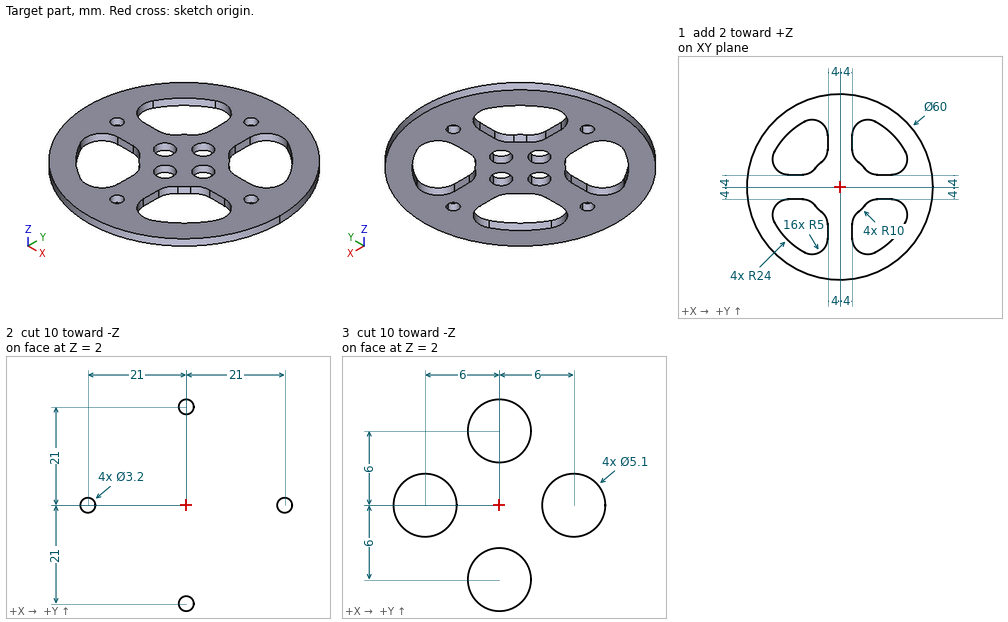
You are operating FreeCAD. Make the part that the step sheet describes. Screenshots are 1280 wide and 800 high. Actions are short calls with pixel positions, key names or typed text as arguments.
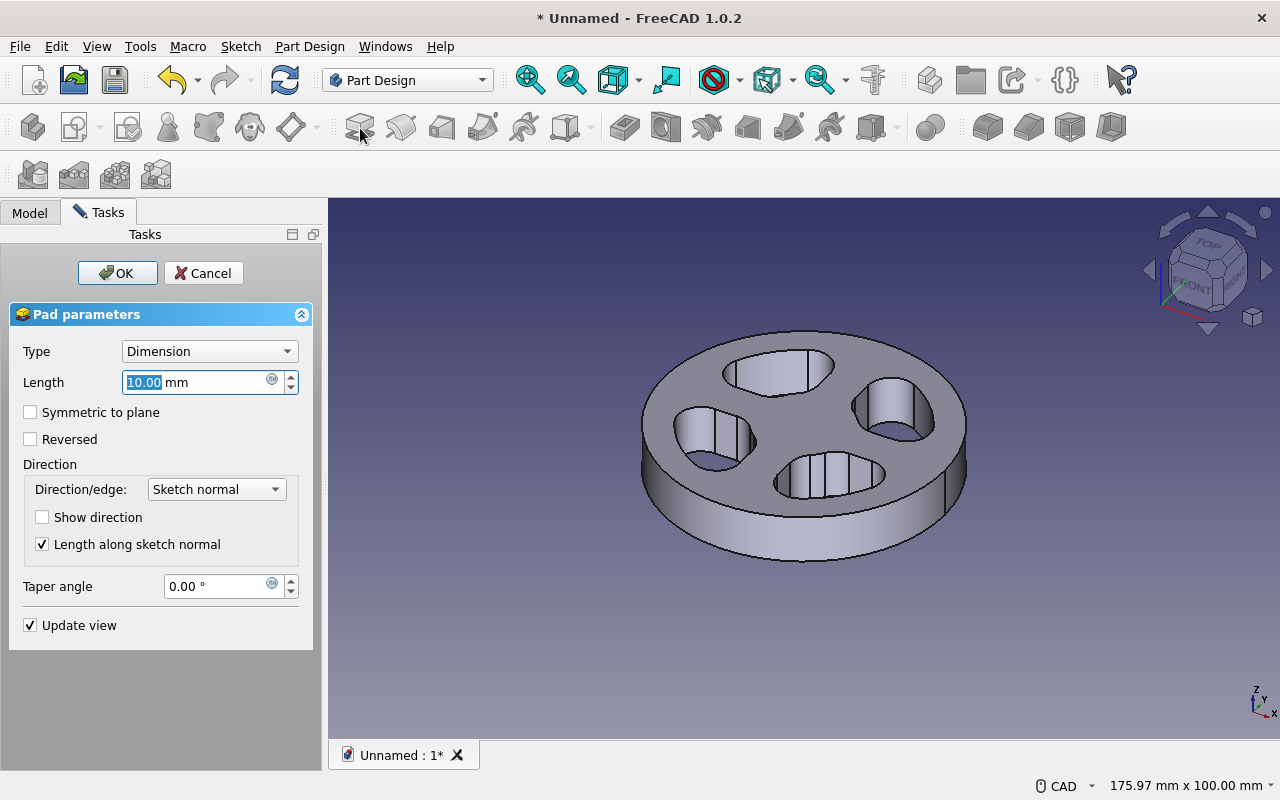
text(2)
key(Tab)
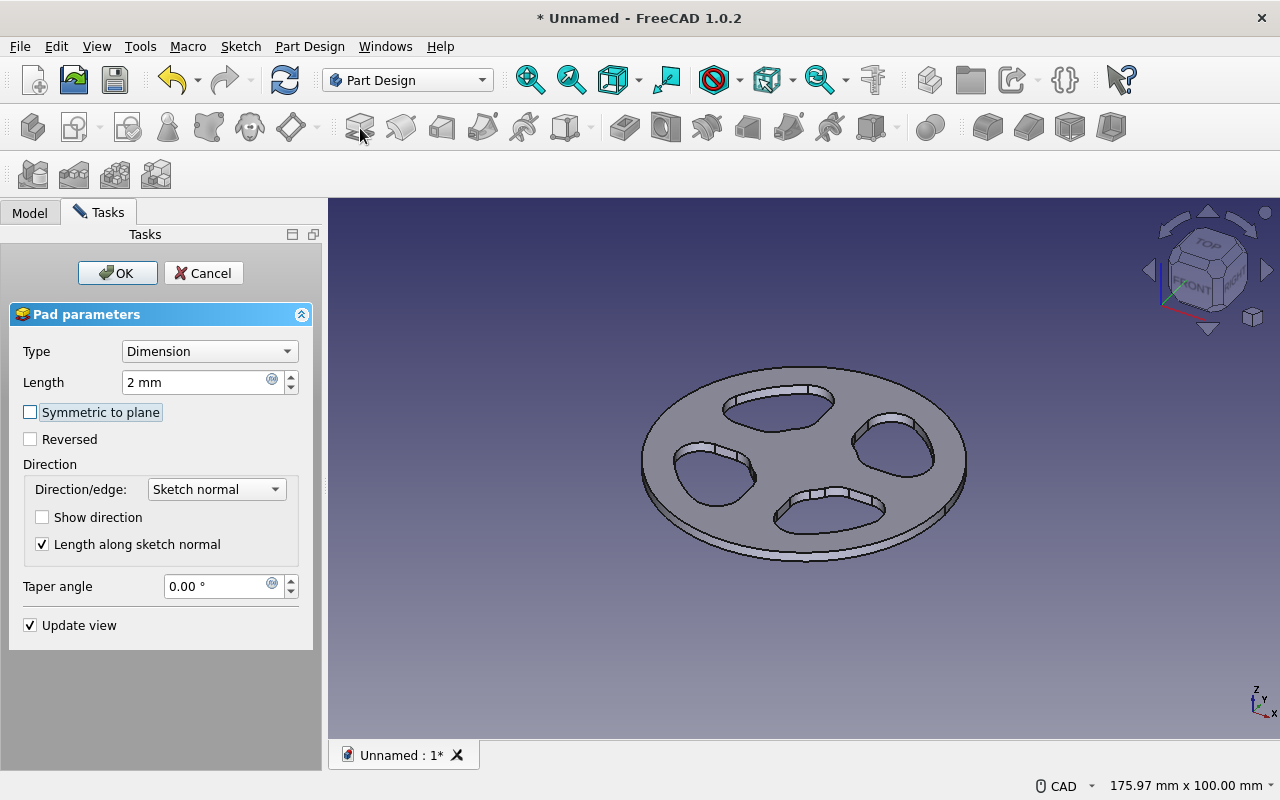
click(118, 273)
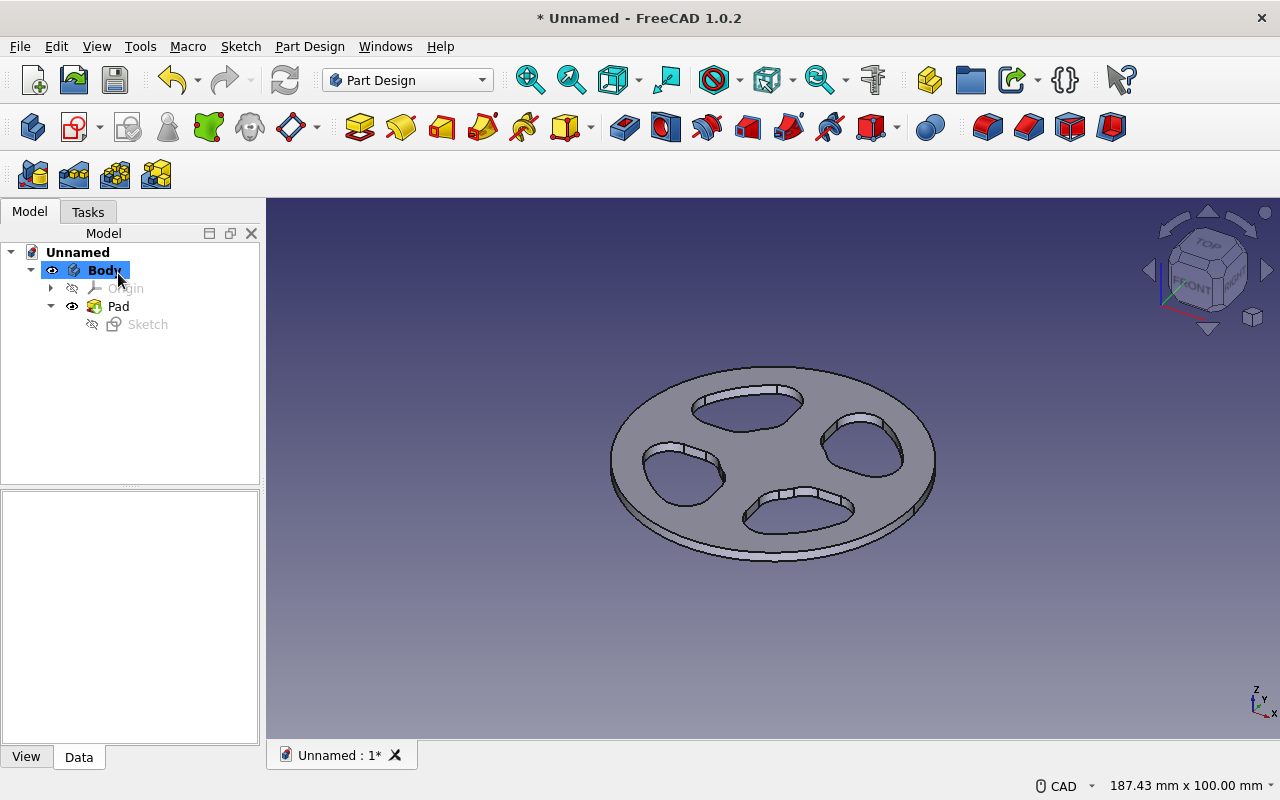
click(773, 459)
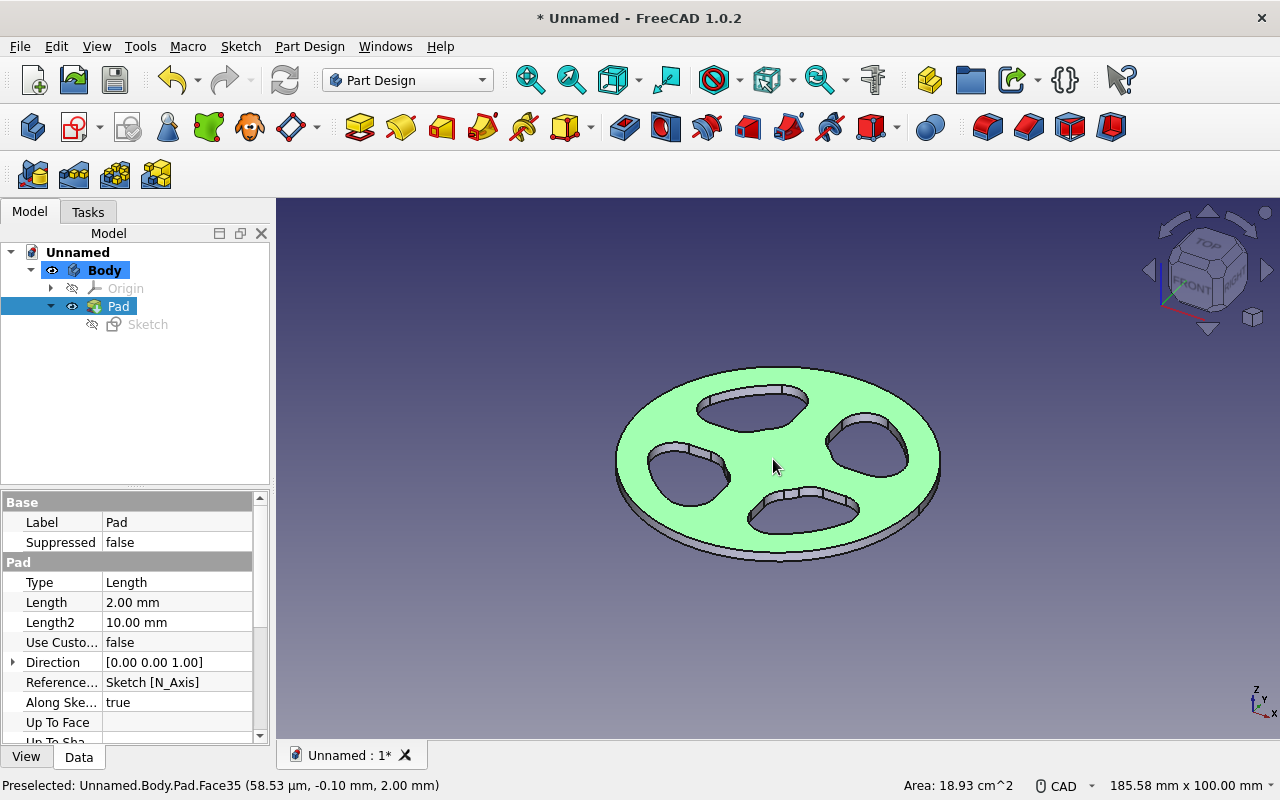
click(74, 128)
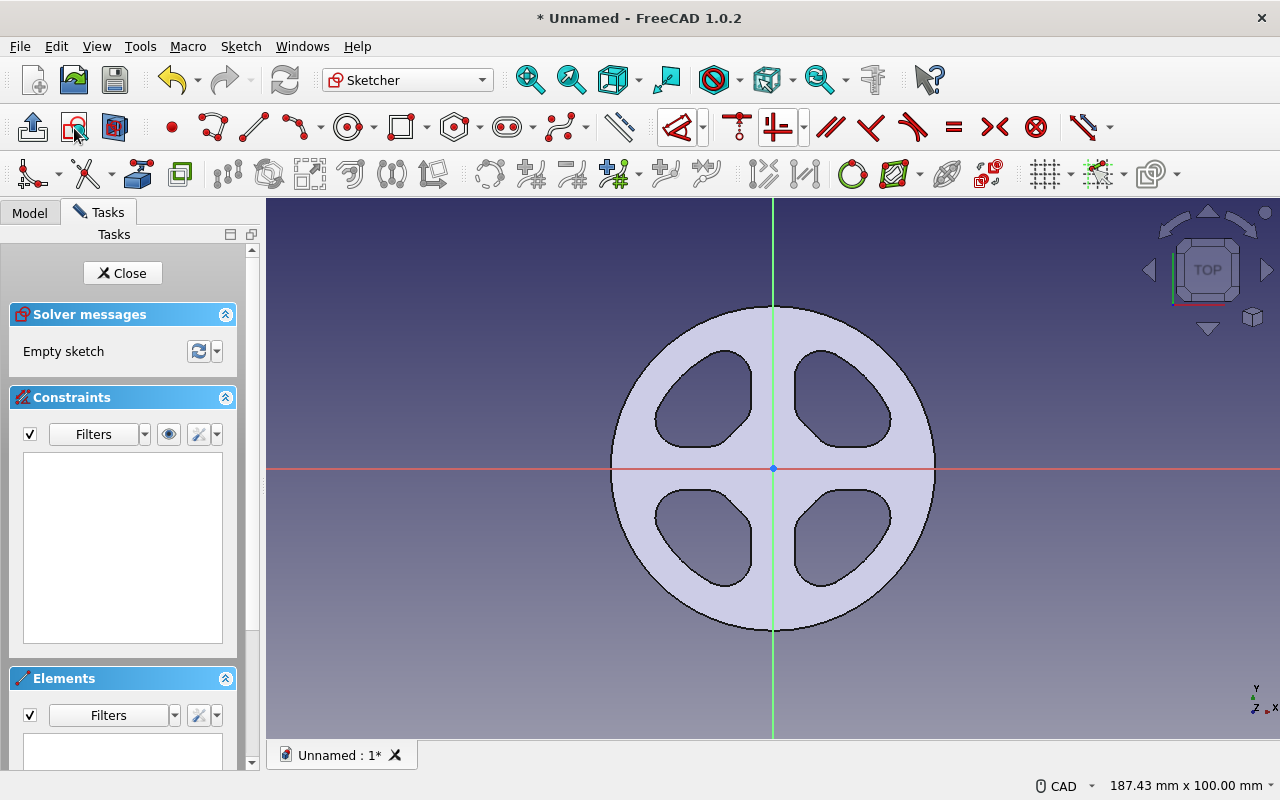
scroll(912, 469, up, 2)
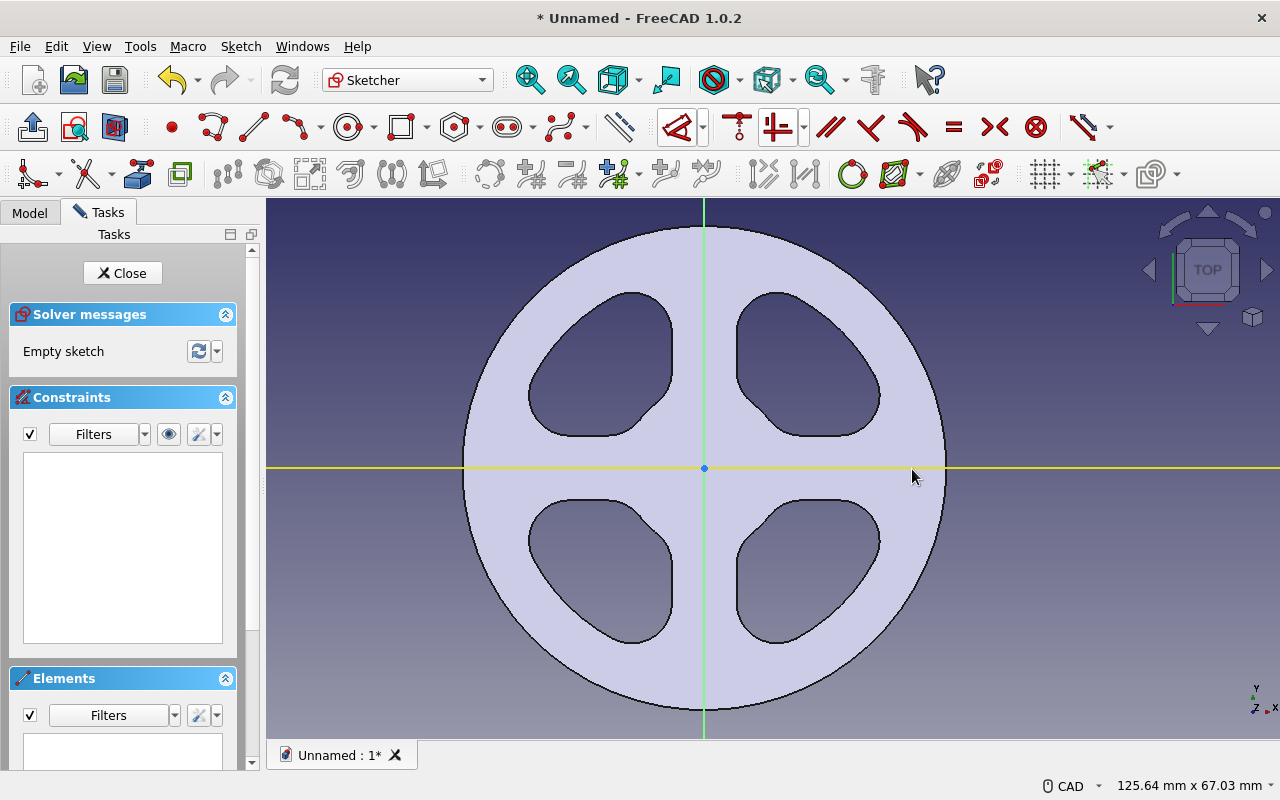
click(348, 128)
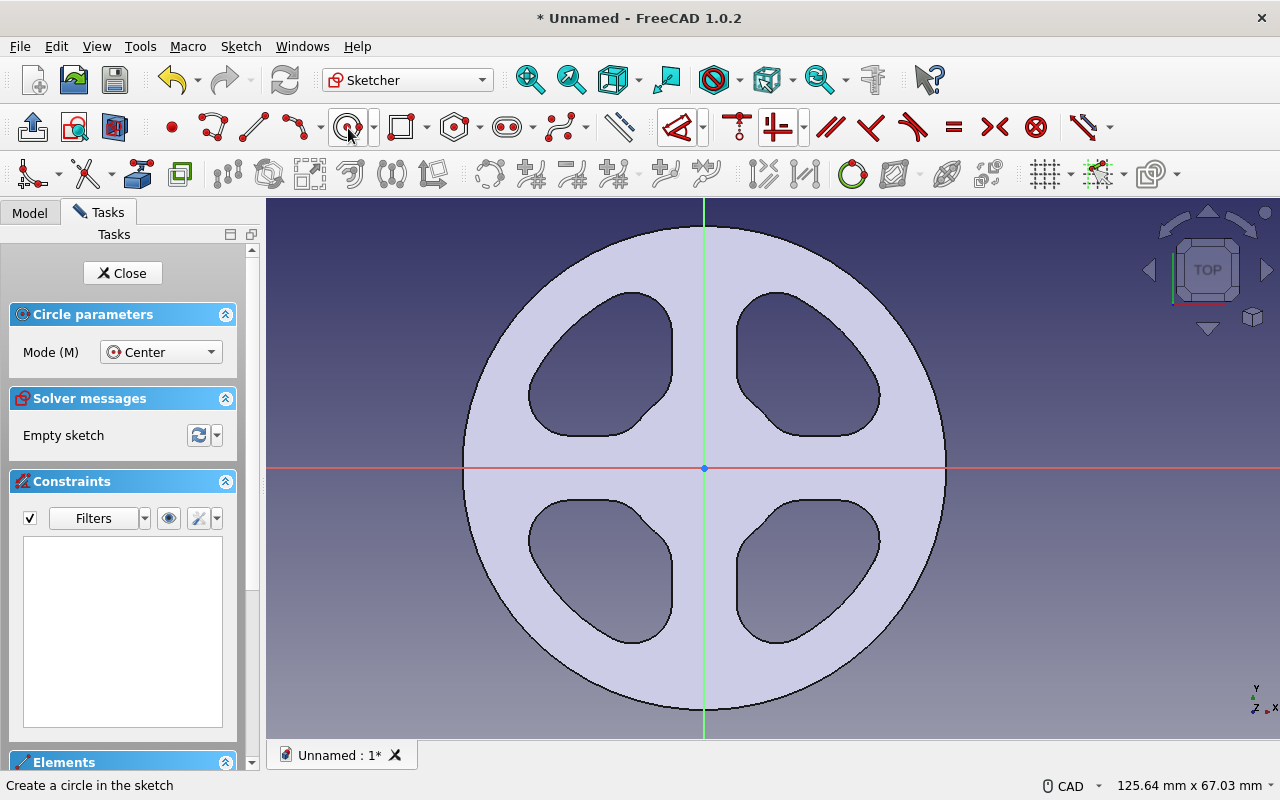
scroll(535, 468, up, 3)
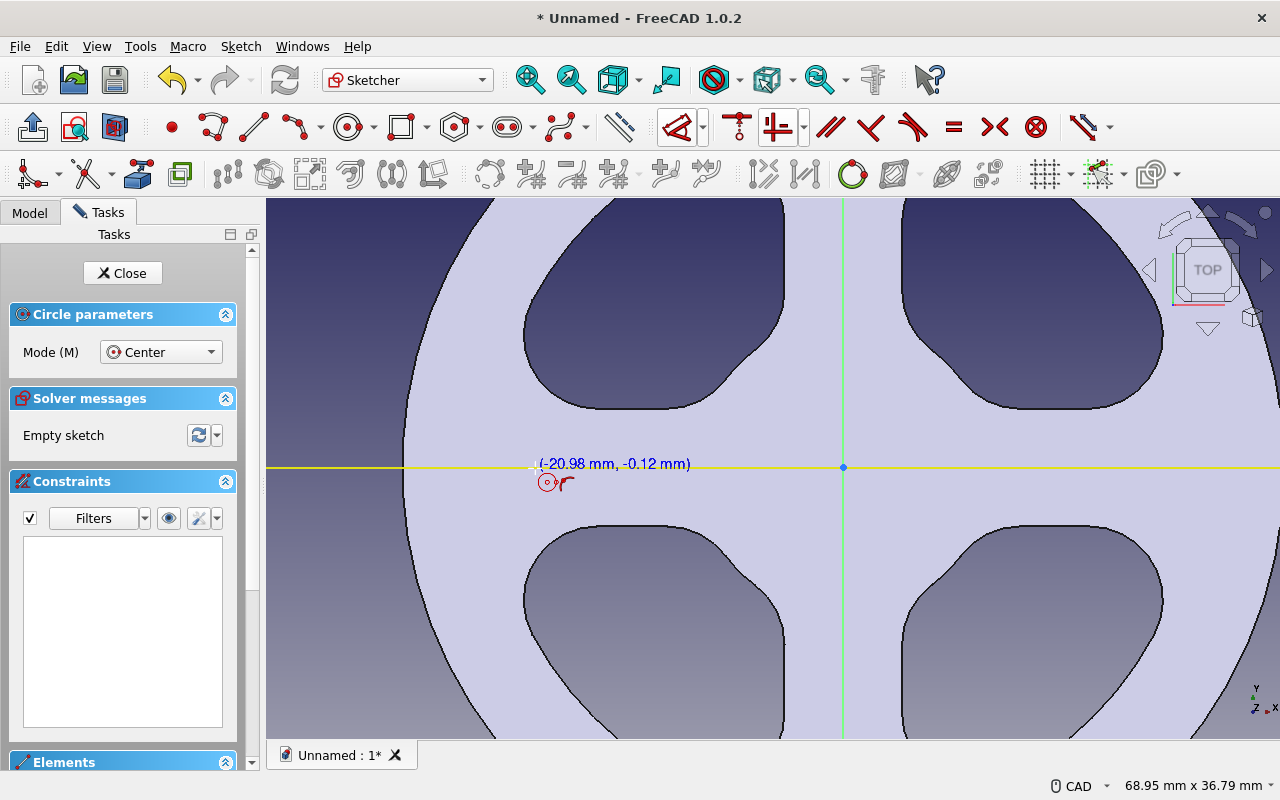
click(534, 468)
move(551, 451)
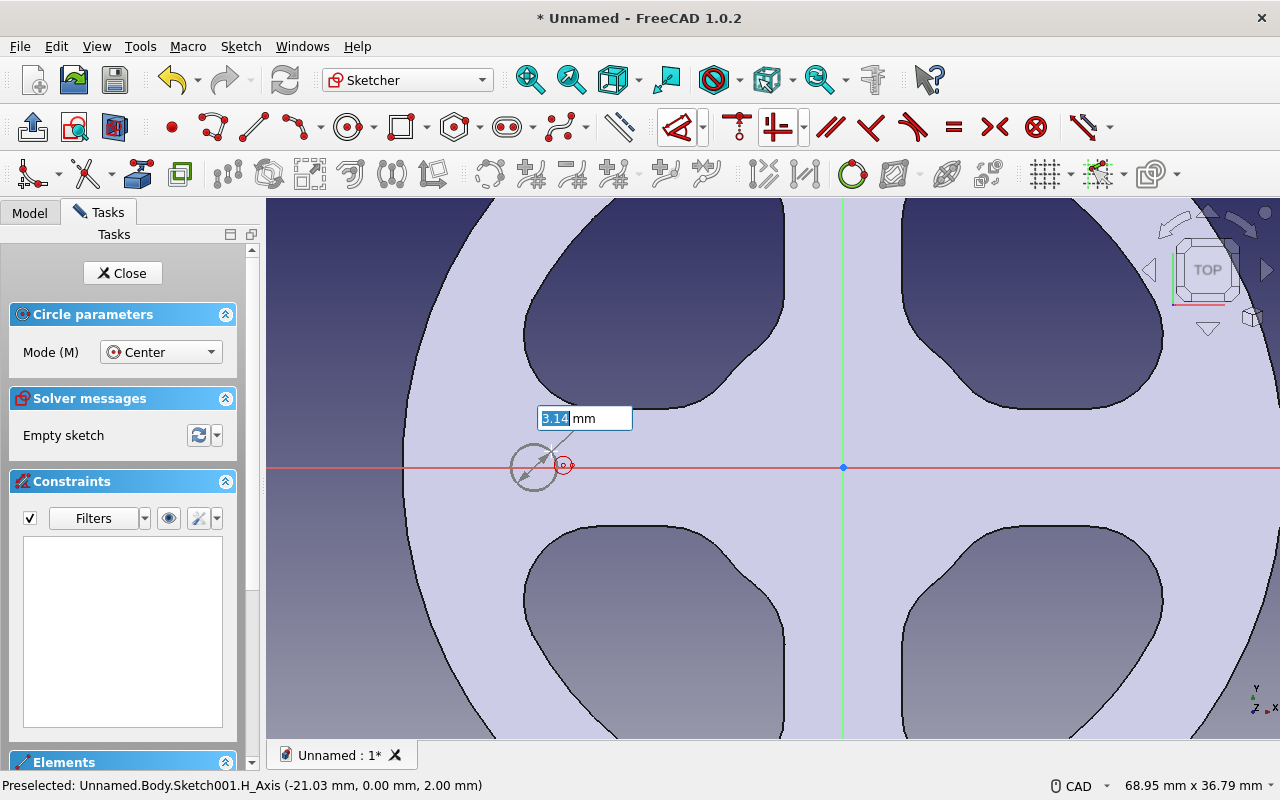
text(3.2)
key(Return)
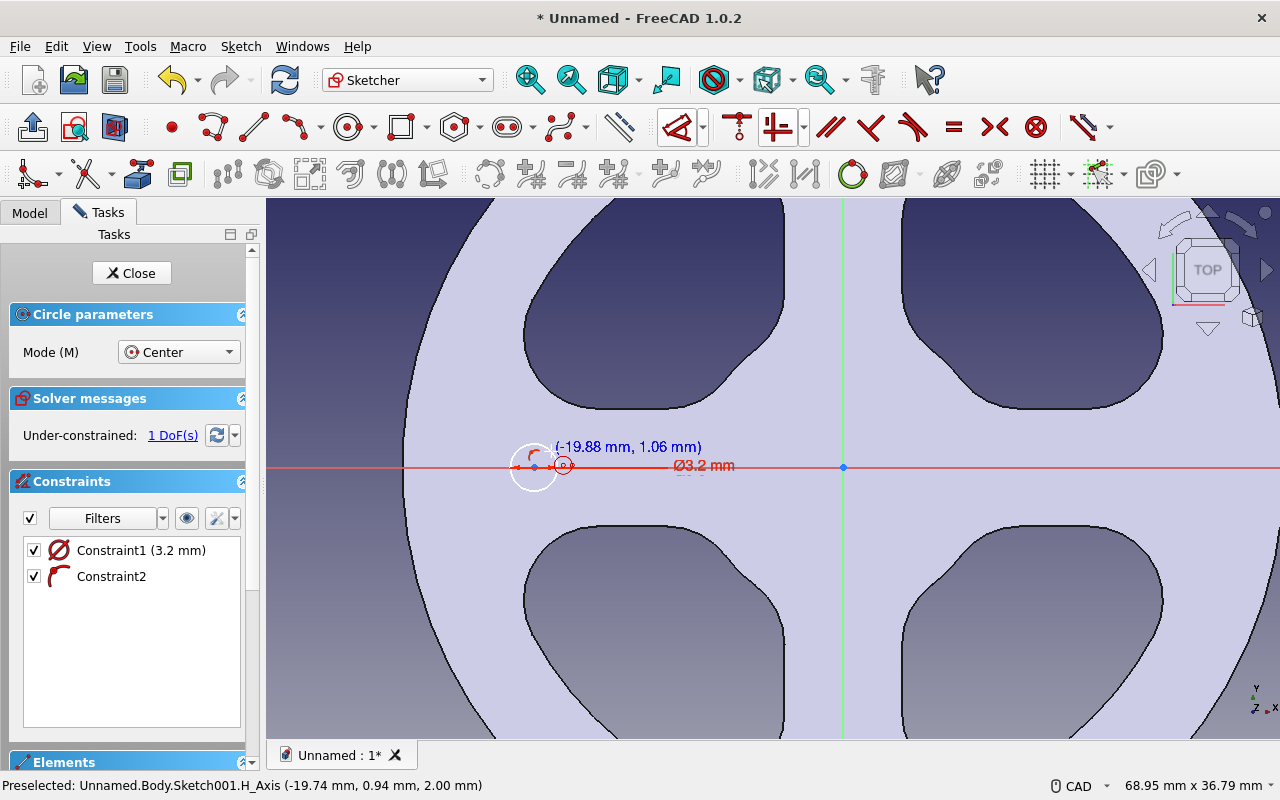
scroll(536, 470, down, 3)